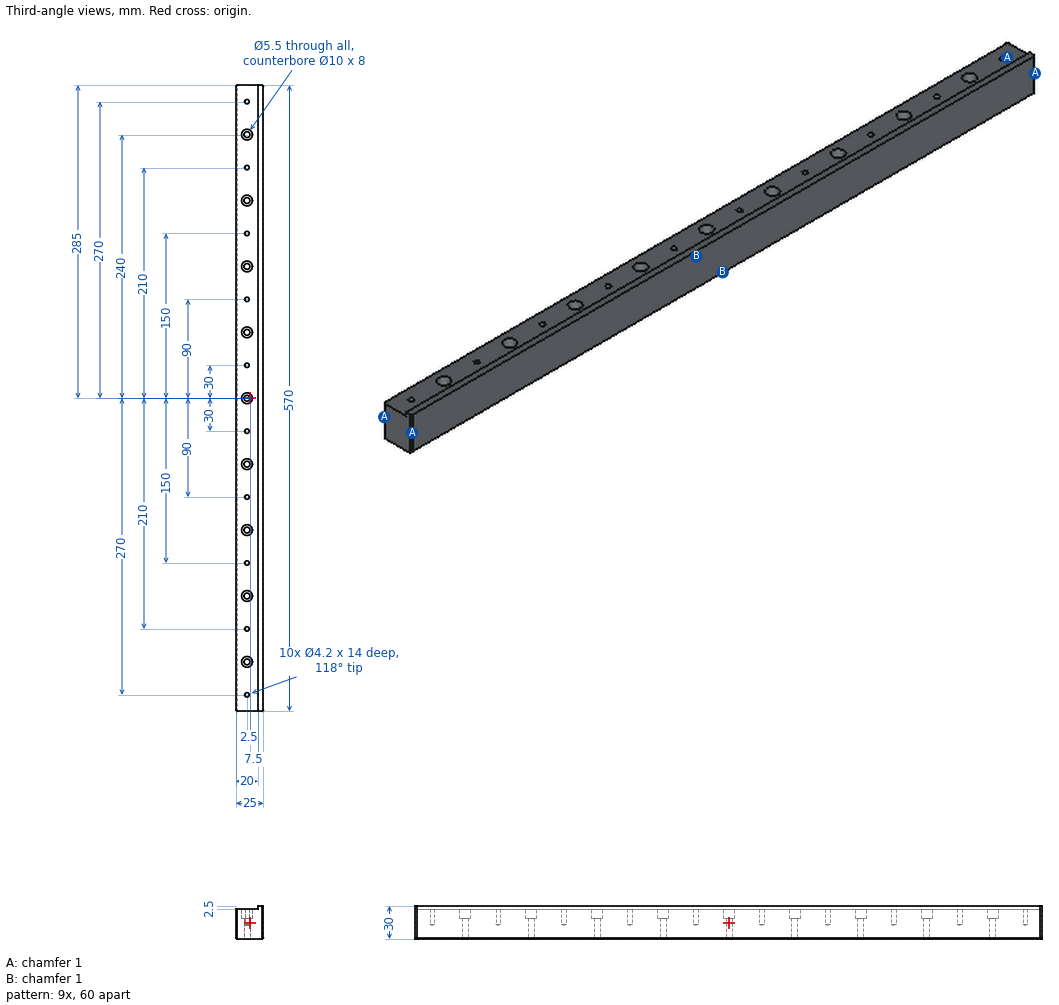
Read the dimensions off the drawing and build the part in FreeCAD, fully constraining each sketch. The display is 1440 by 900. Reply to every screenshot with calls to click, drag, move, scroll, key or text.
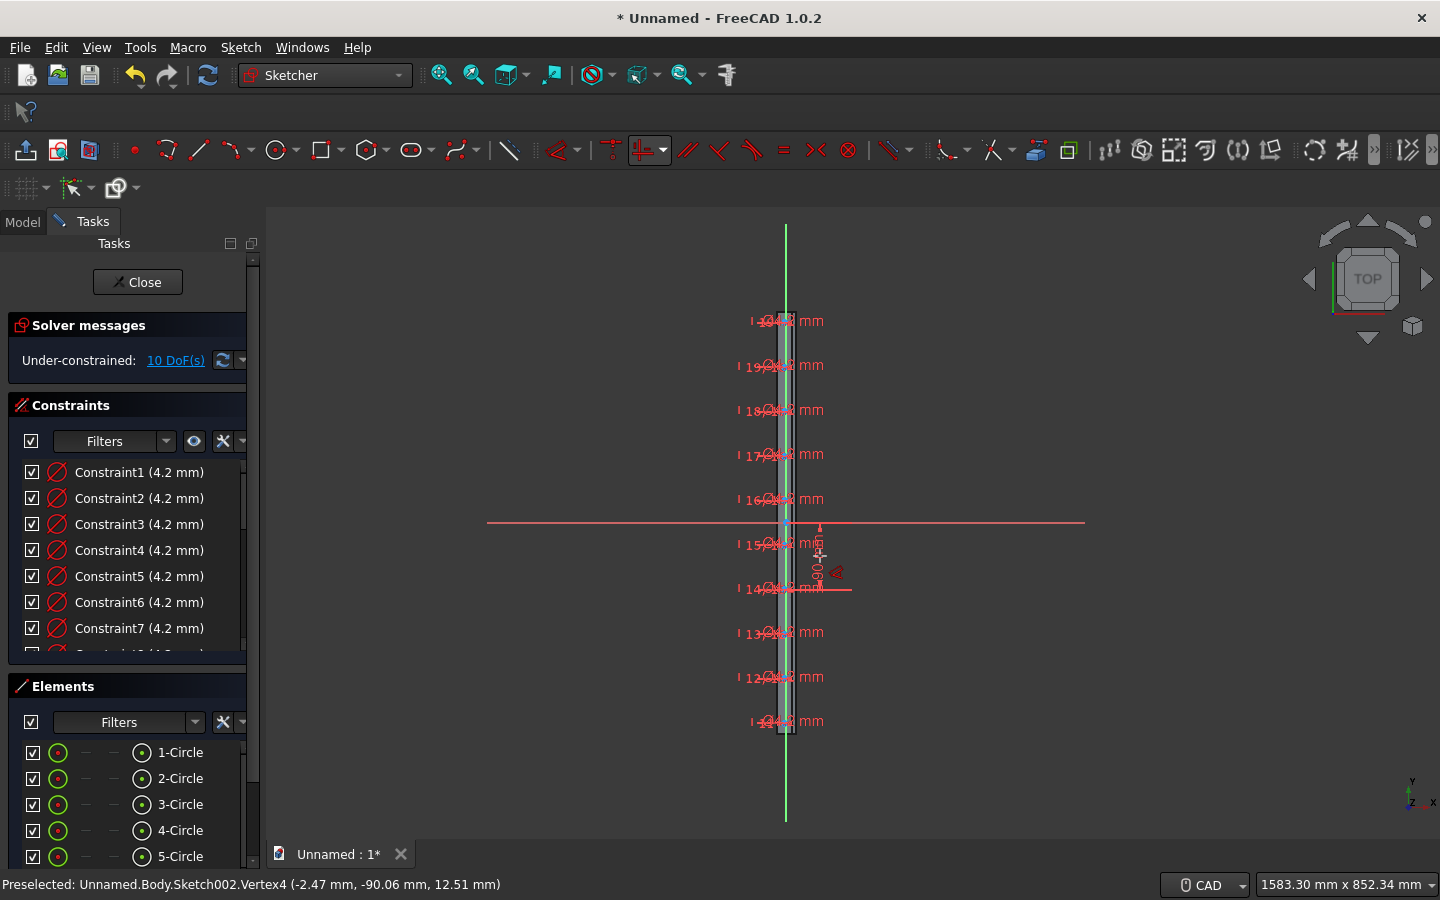
scroll(785, 545, up, 3)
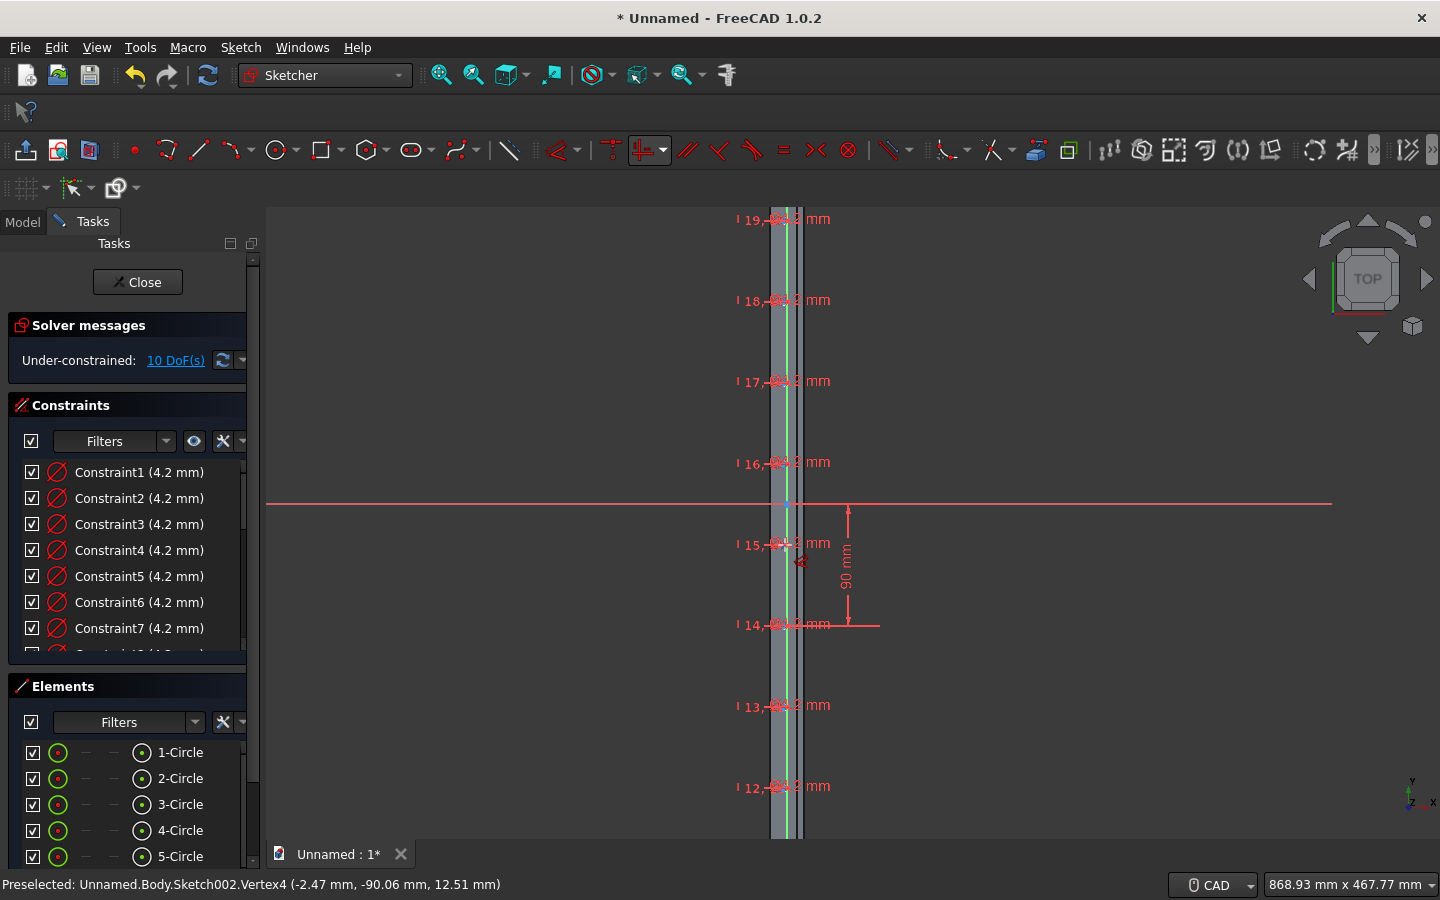
click(784, 545)
click(821, 525)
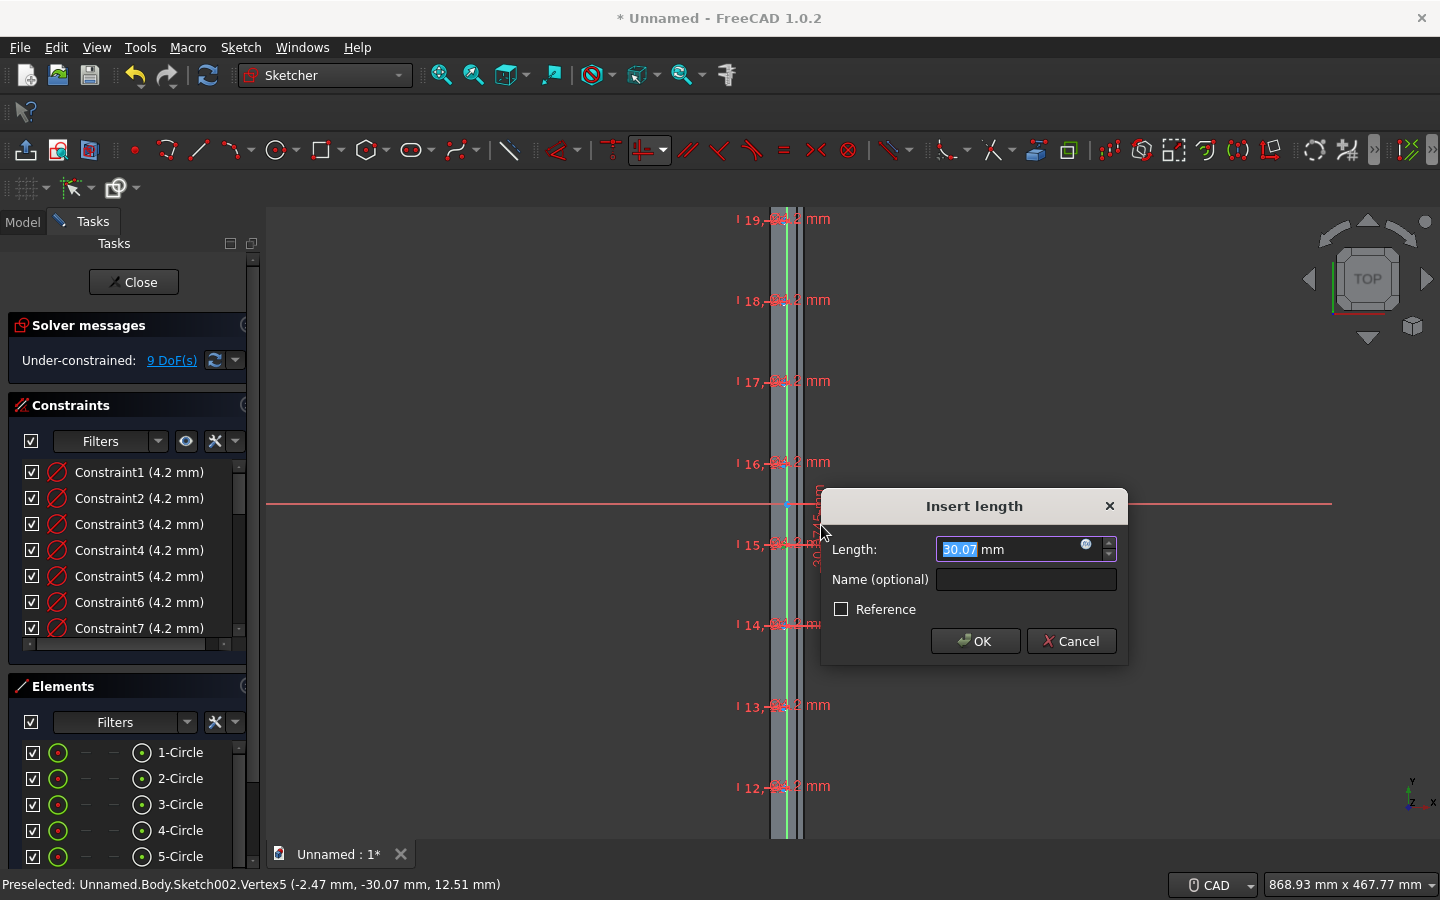
text(30)
key(Return)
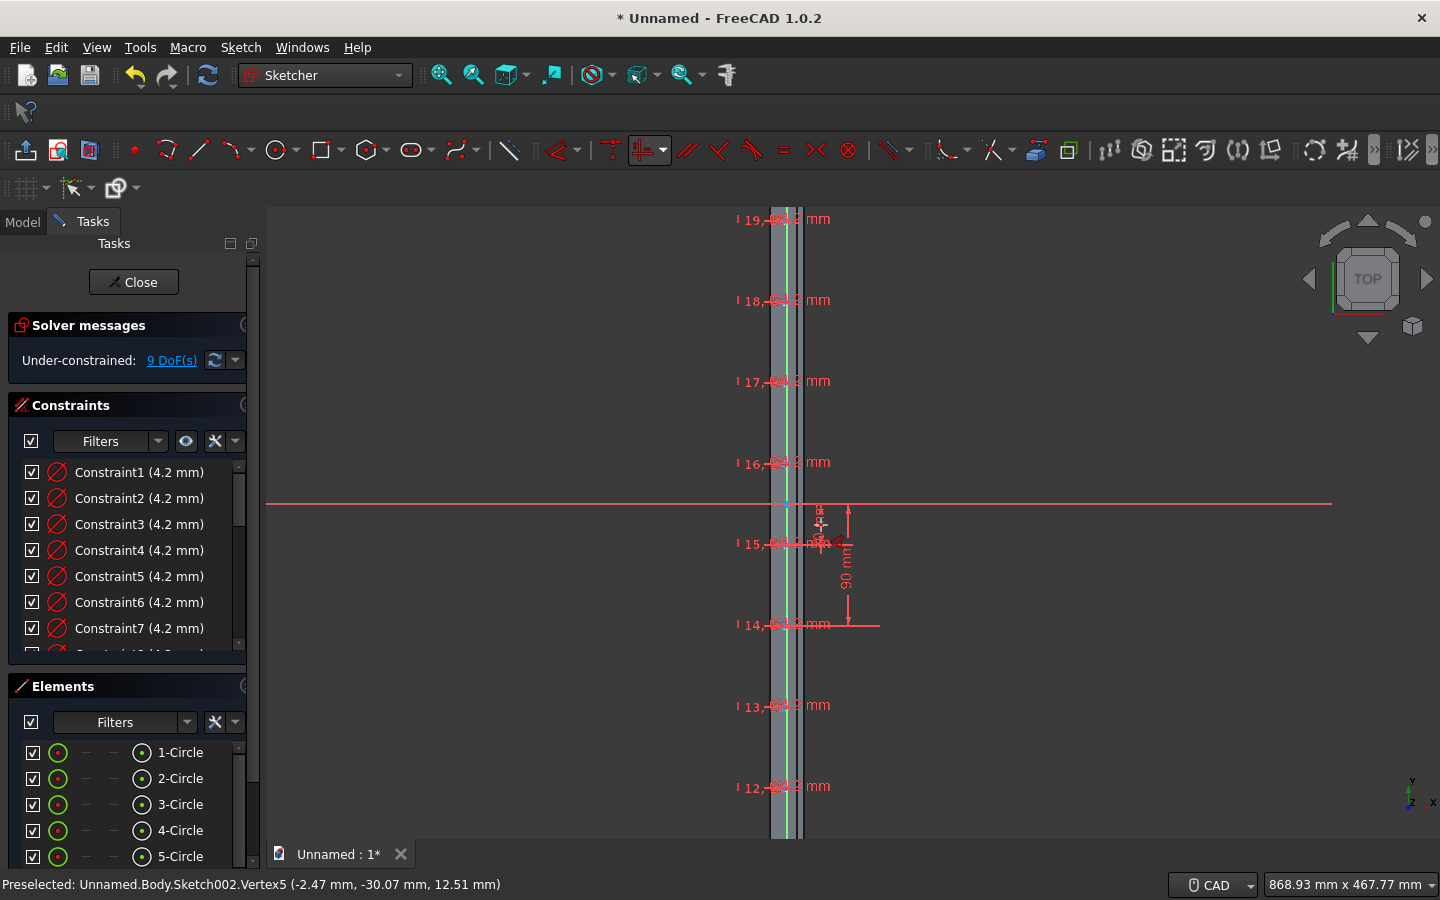
click(784, 464)
click(821, 484)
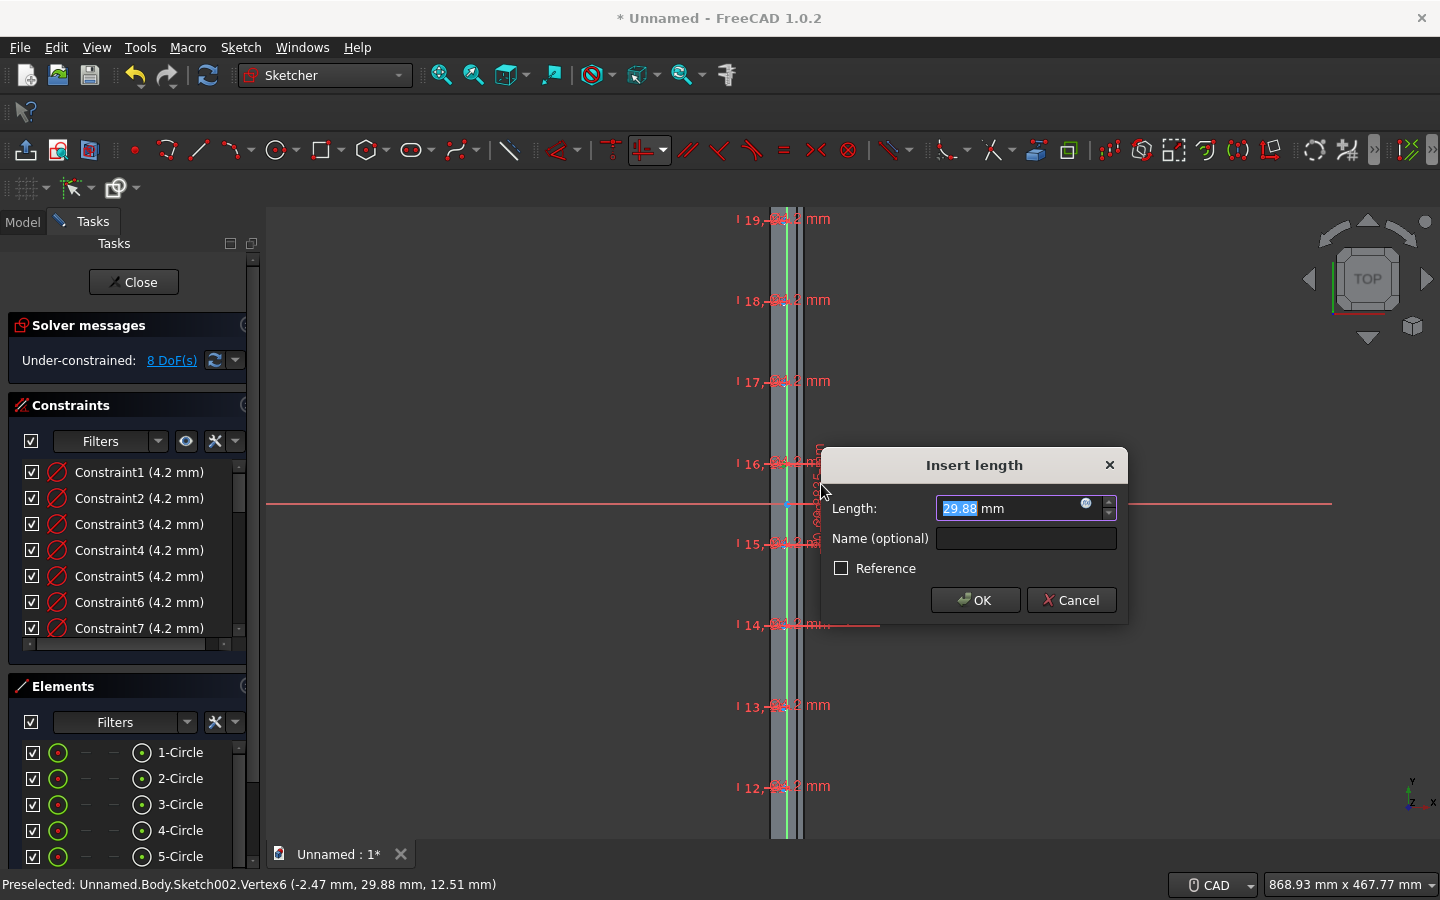
text(30)
key(Return)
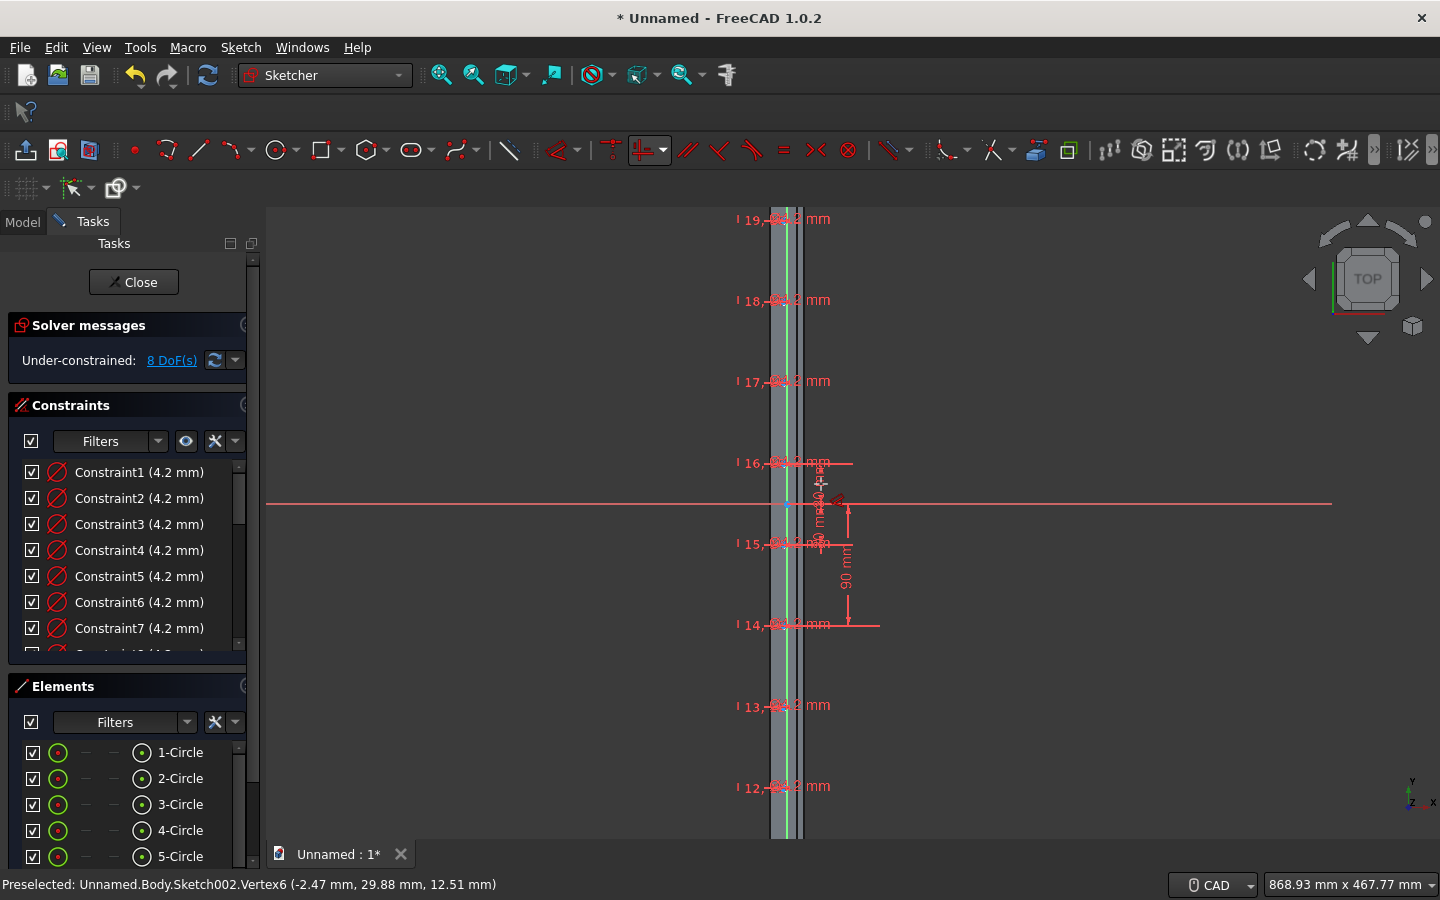
click(784, 383)
click(821, 444)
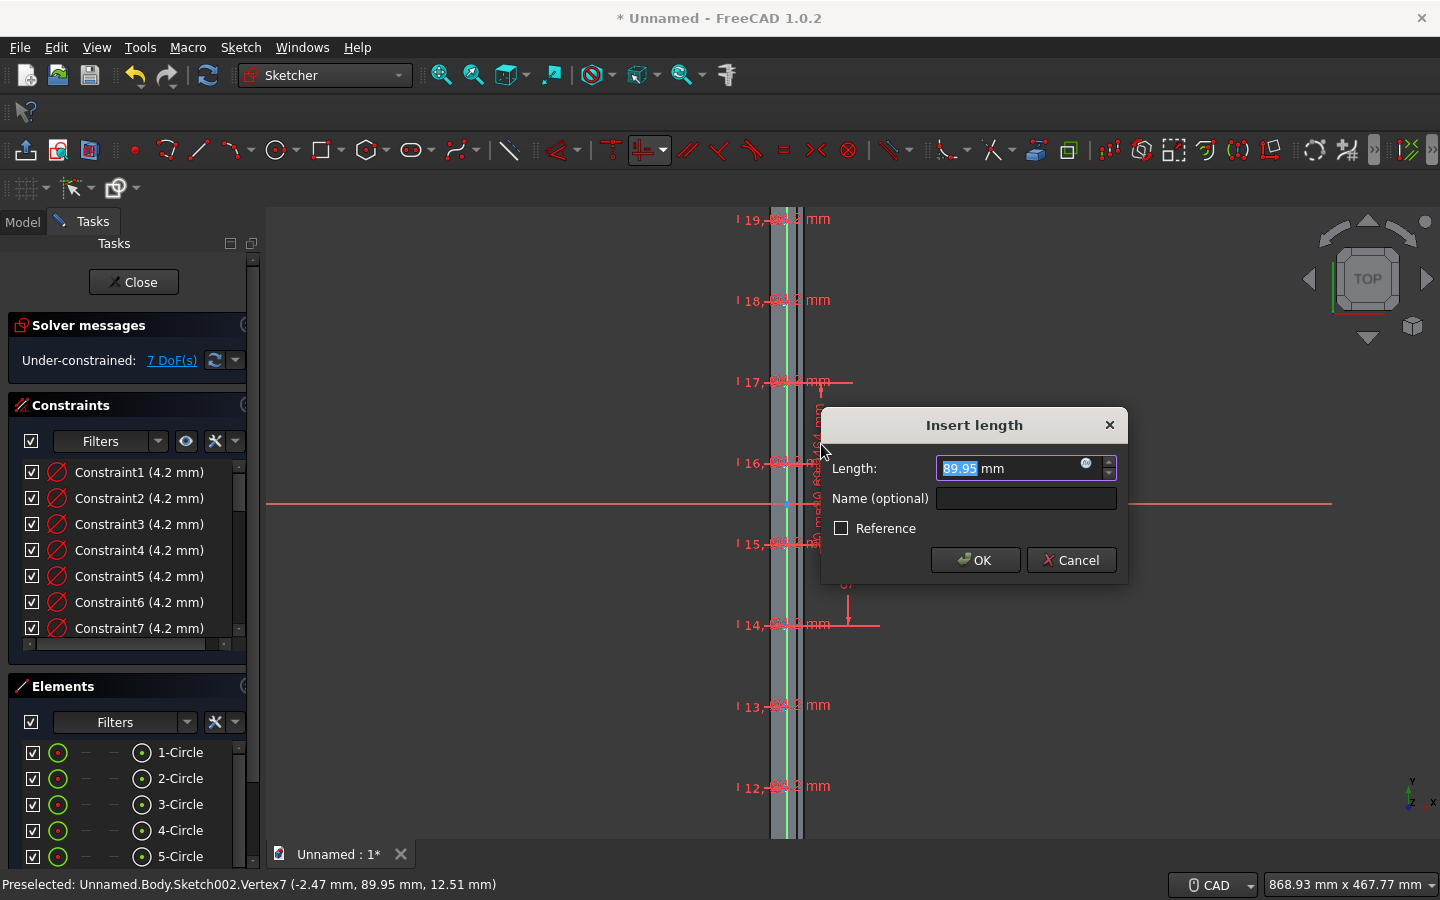
text(90)
key(Return)